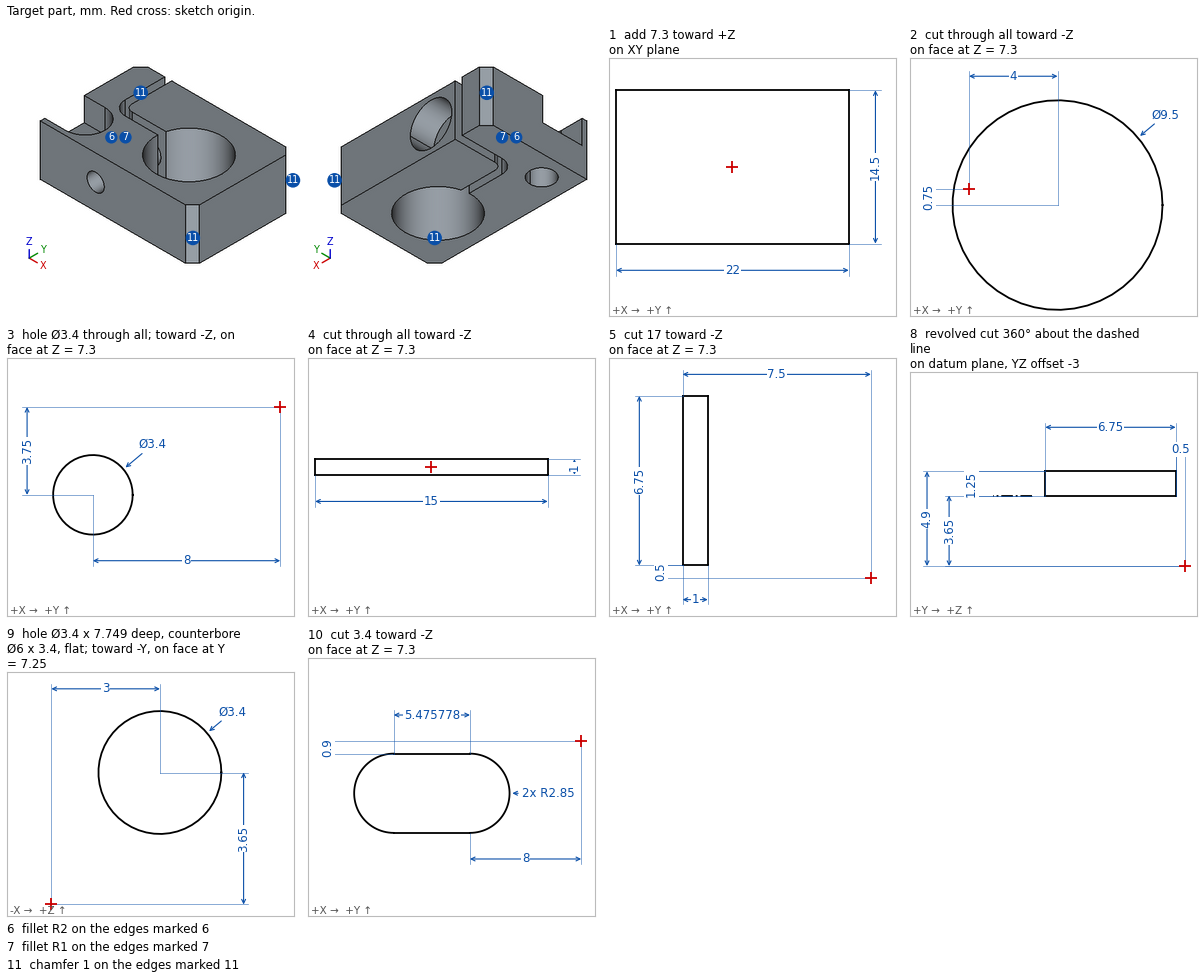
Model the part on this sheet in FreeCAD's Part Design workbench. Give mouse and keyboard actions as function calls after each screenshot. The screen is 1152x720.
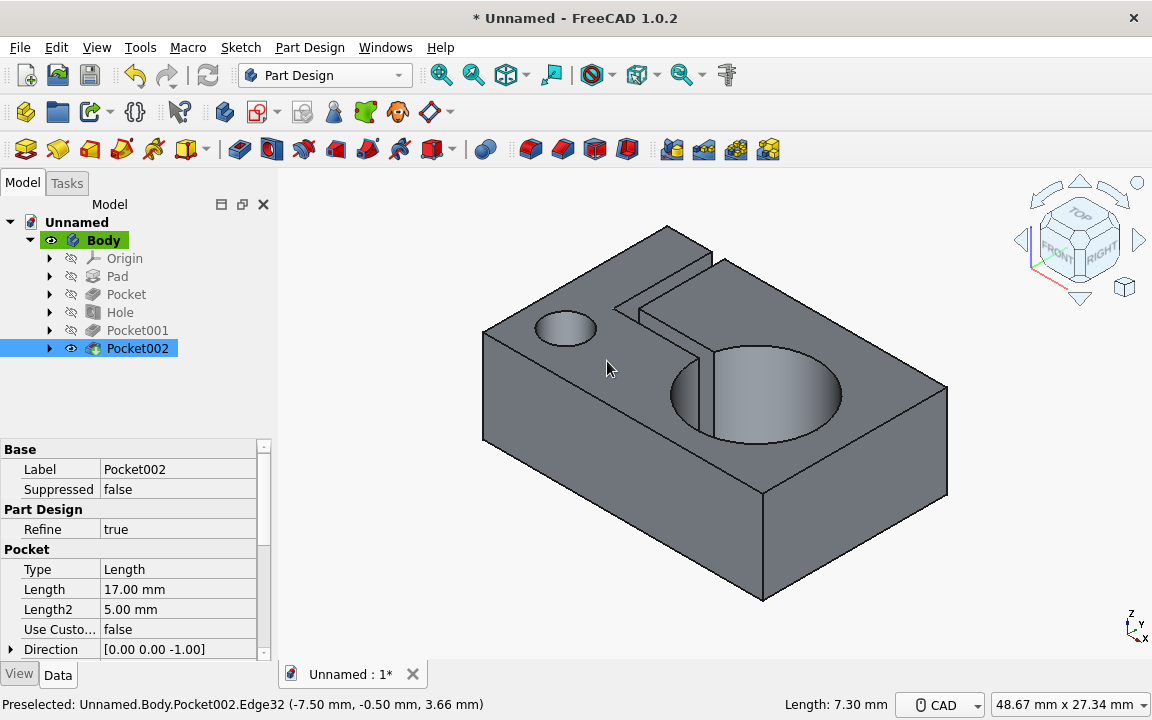
click(532, 150)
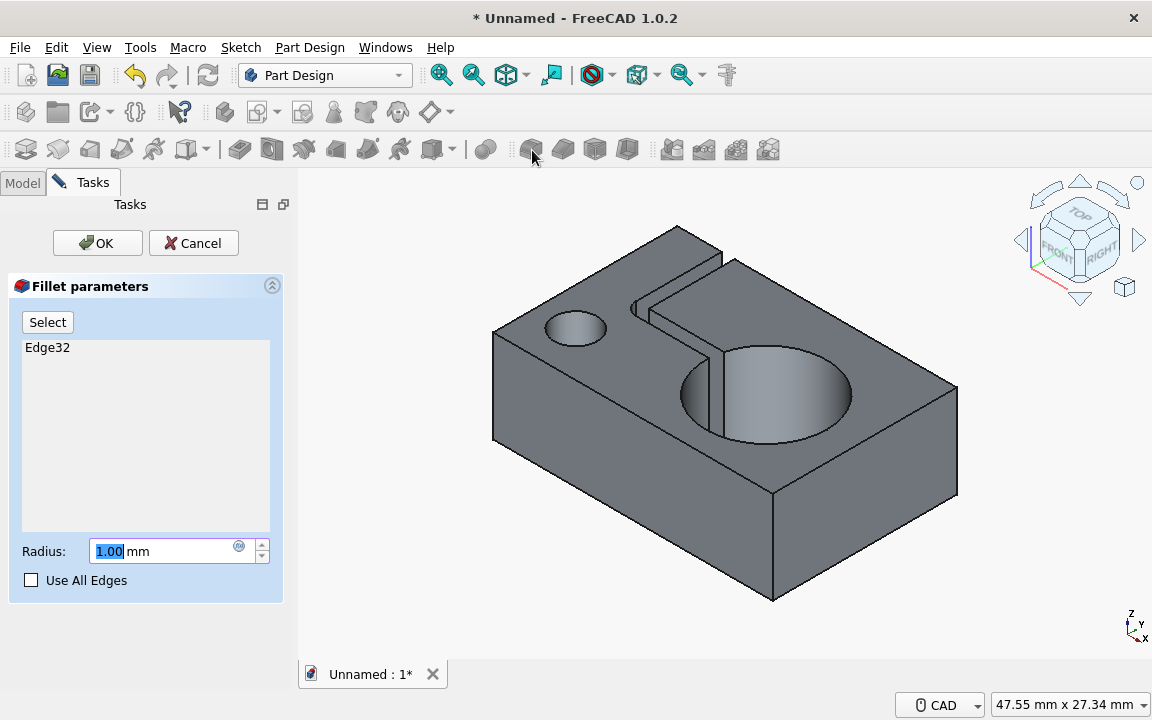
text(2)
key(Tab)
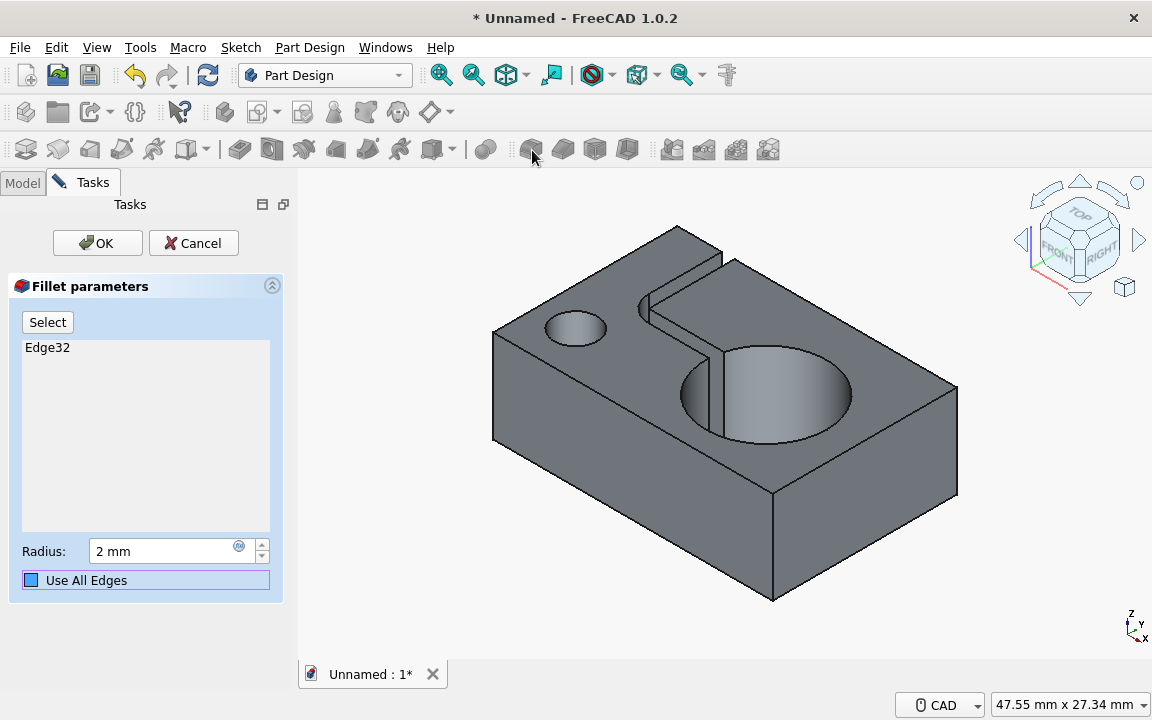
click(98, 243)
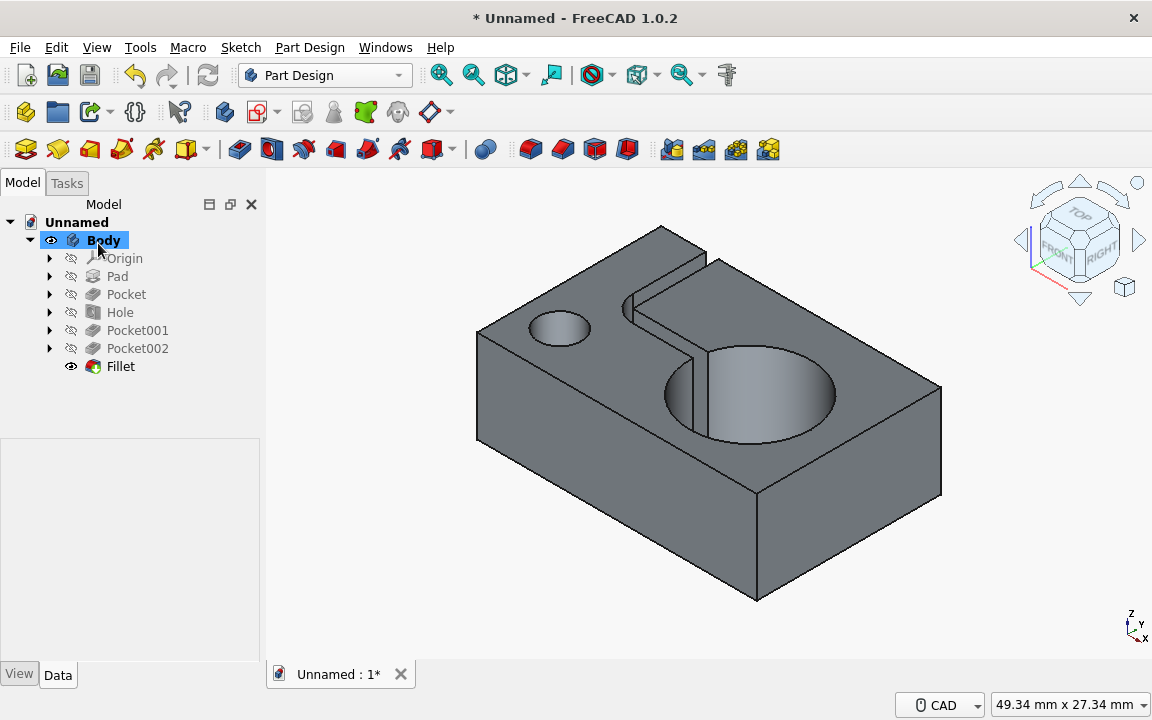
key(2)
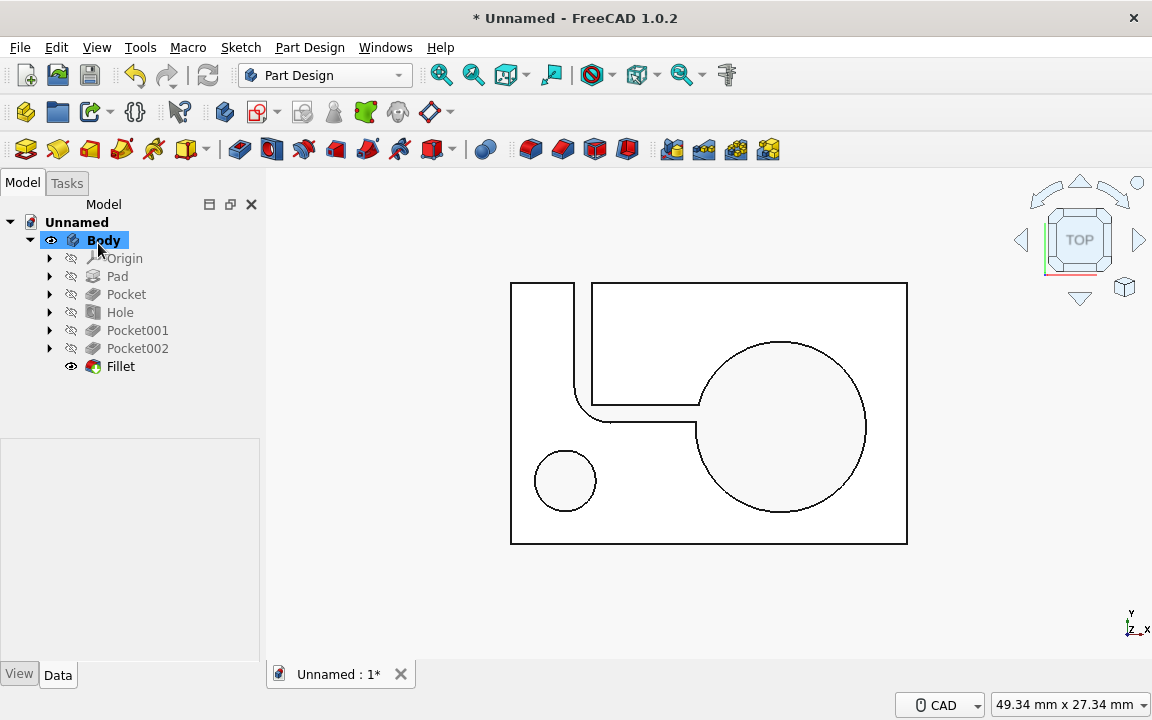
key(0)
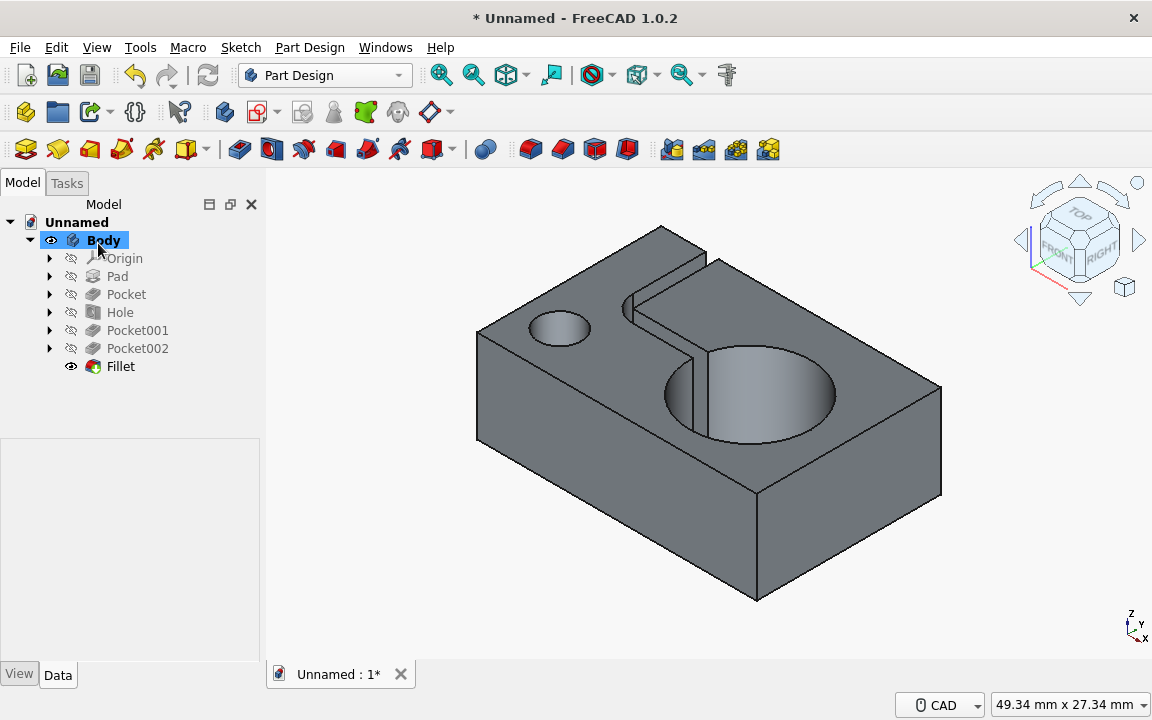
key(1)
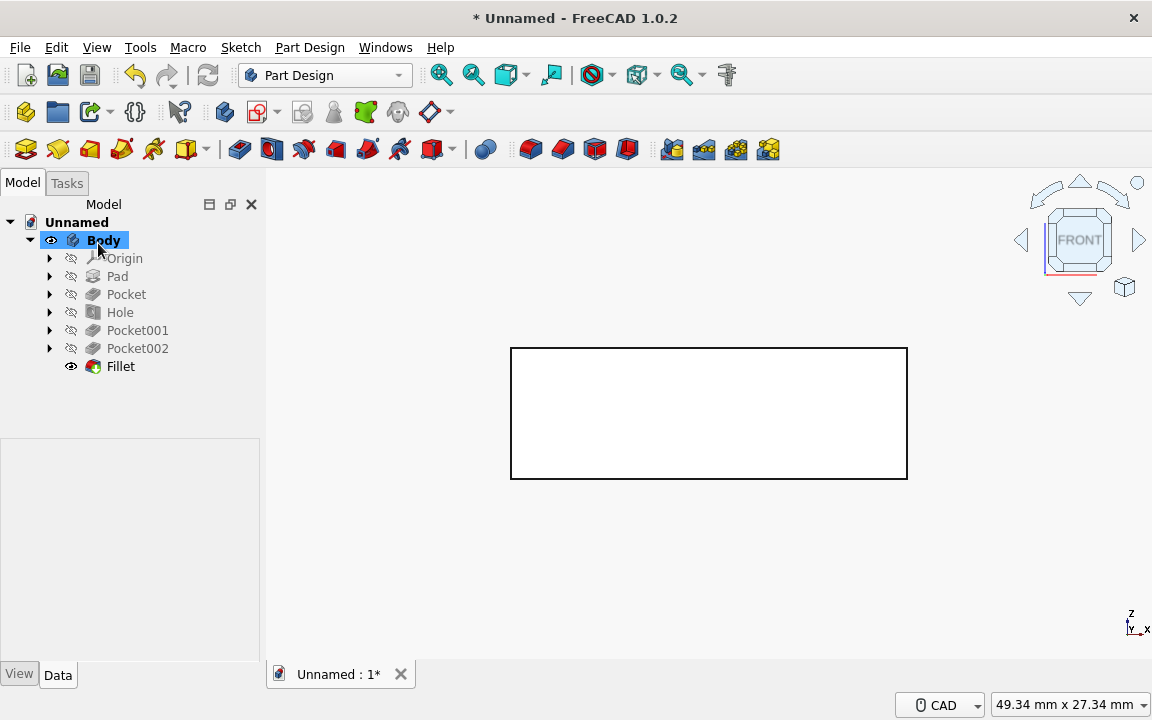
click(442, 76)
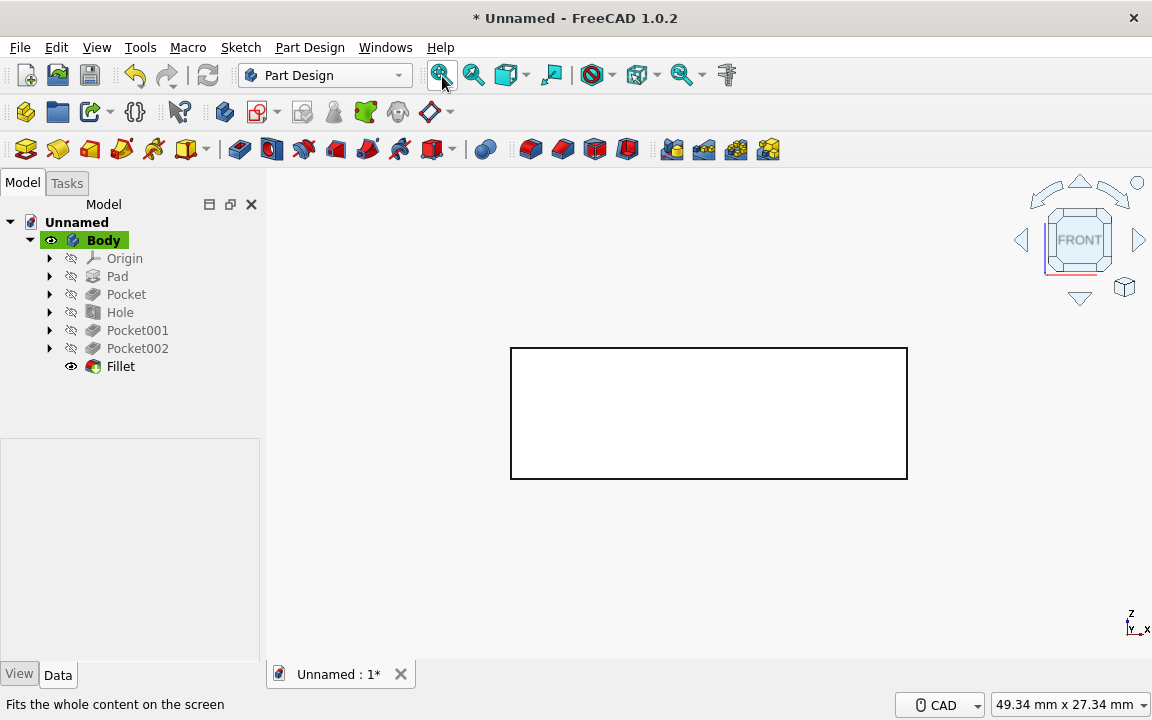
key(3)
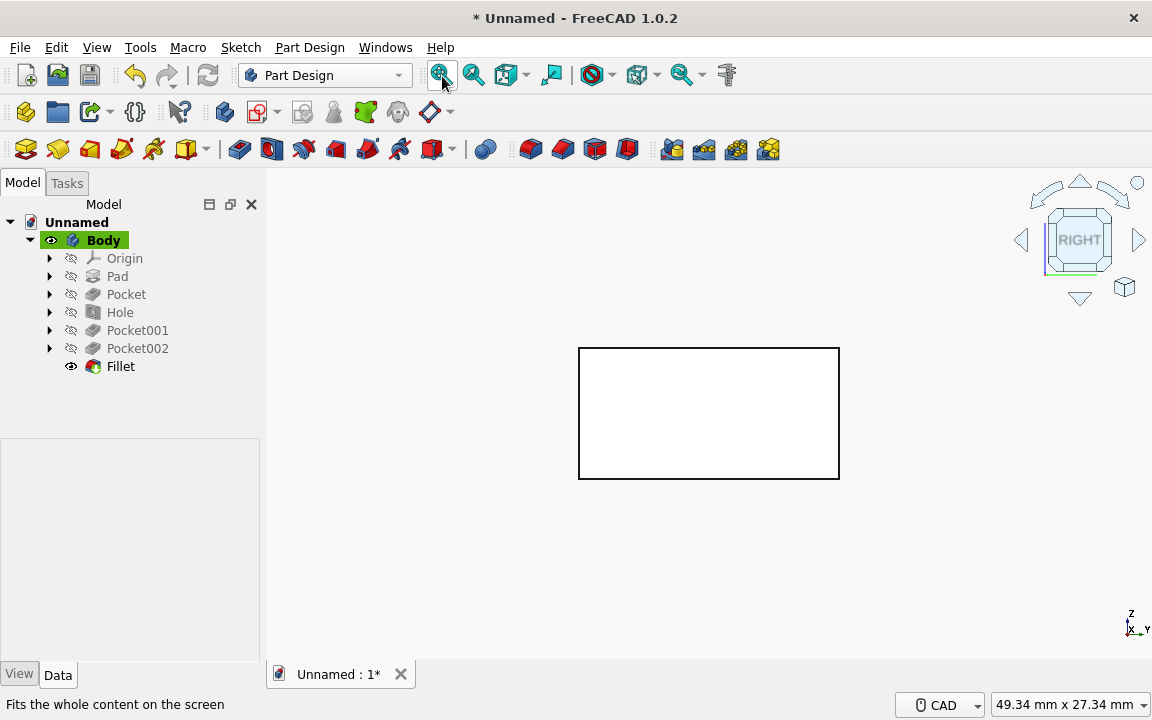
click(442, 76)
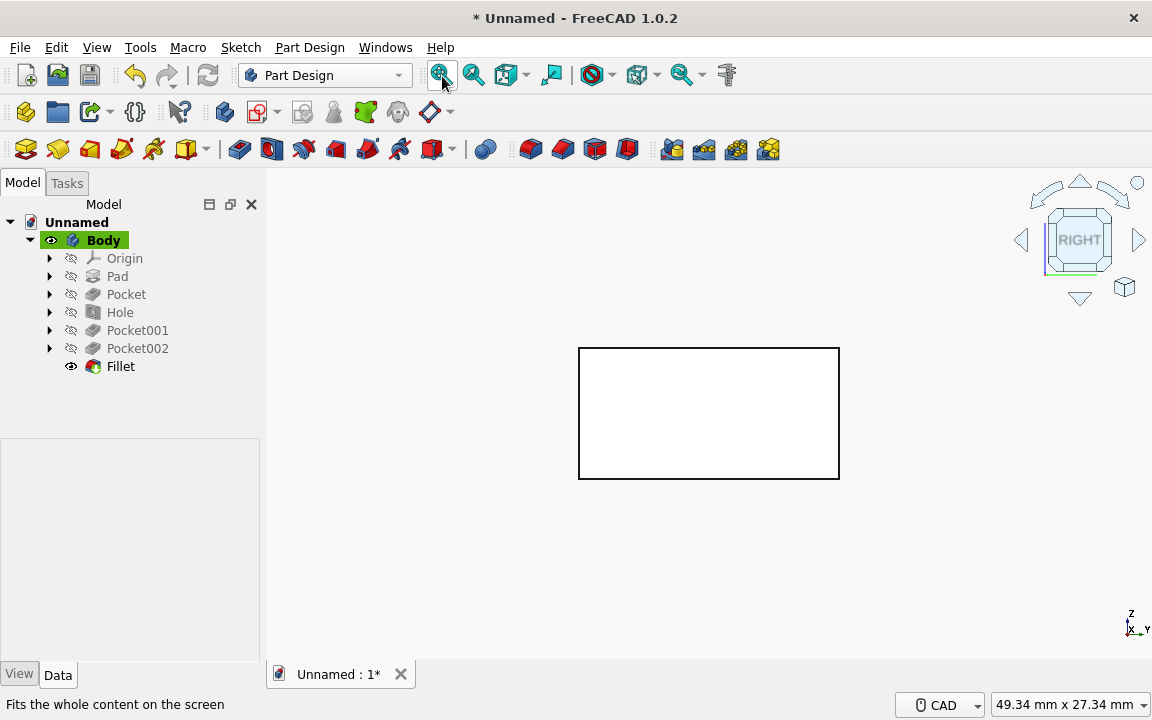
key(5)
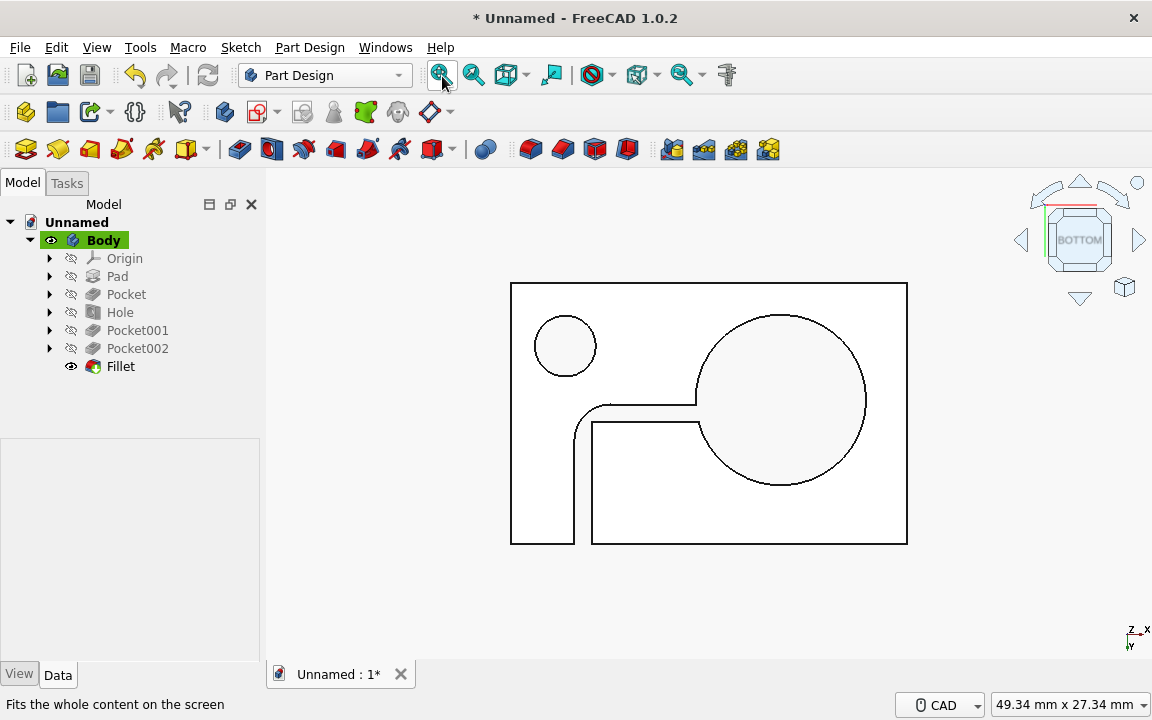
key(4)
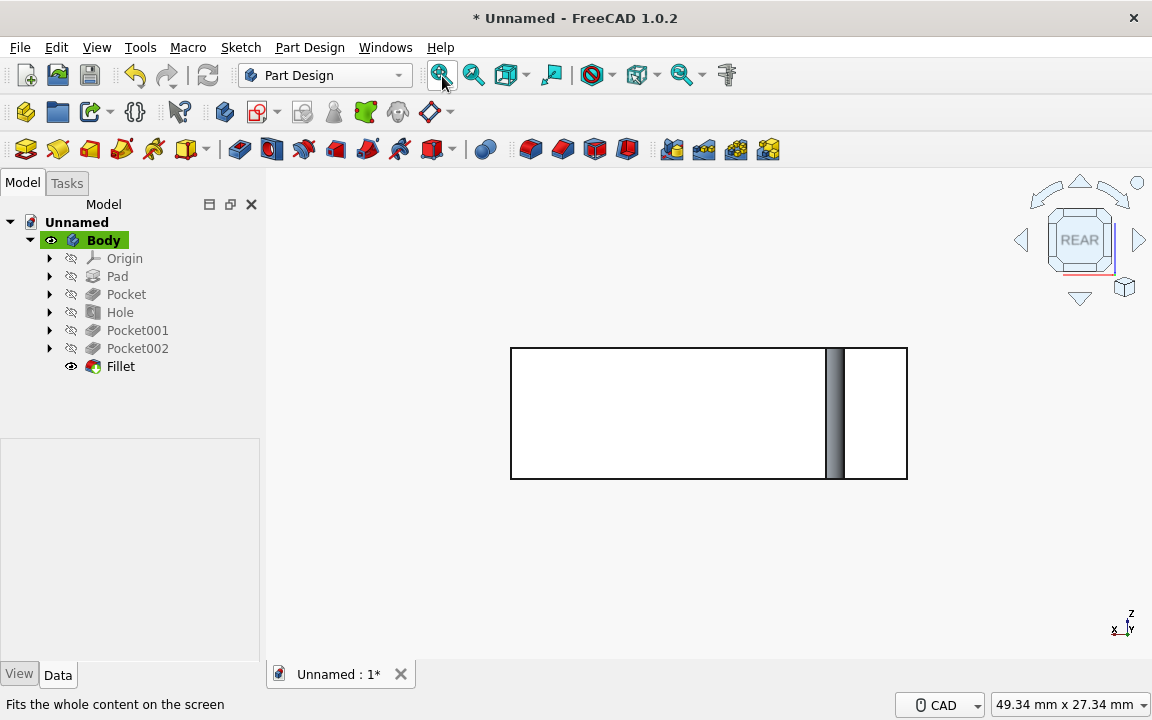
click(442, 76)